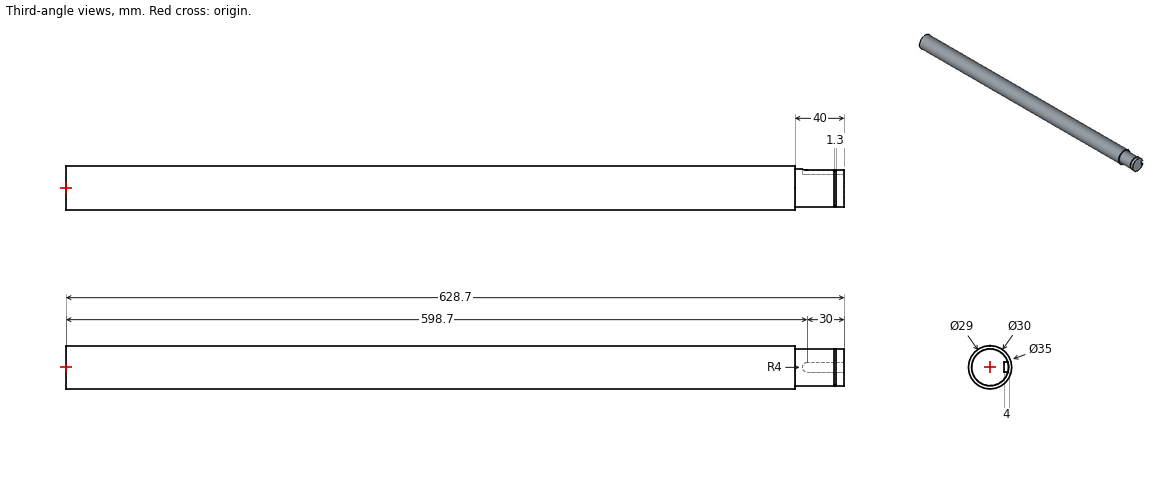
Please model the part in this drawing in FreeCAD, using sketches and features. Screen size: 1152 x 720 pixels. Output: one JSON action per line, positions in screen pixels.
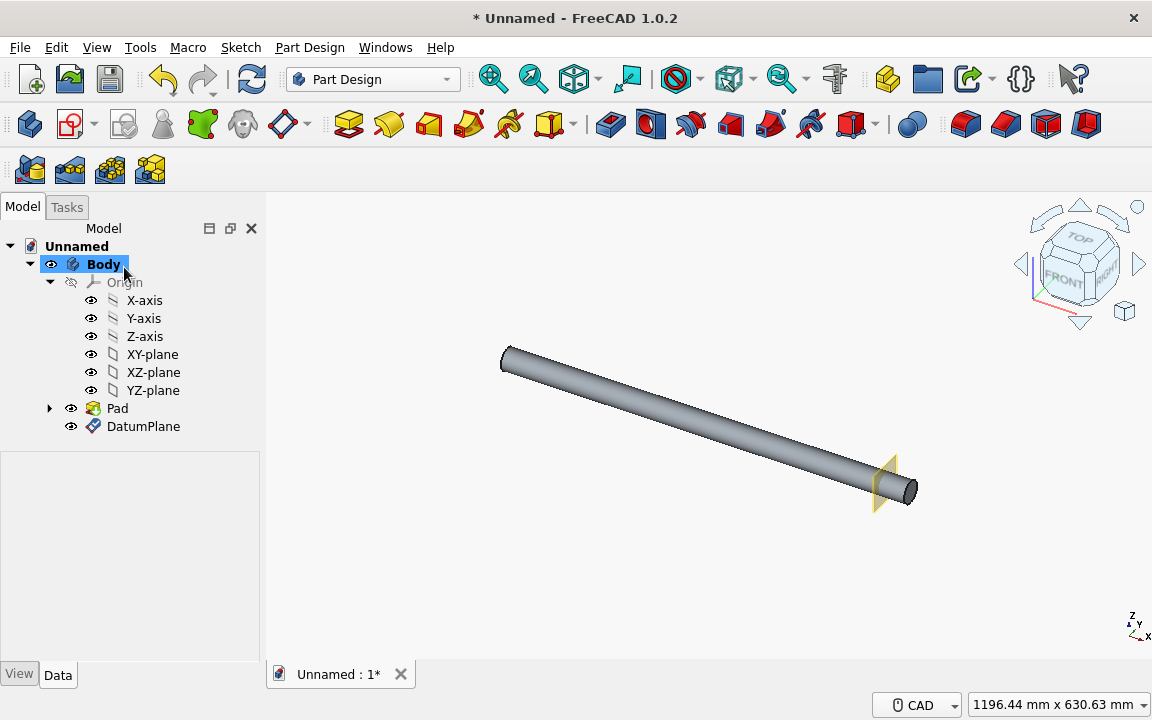
{"action": "left_click", "coordinate": [116, 426]}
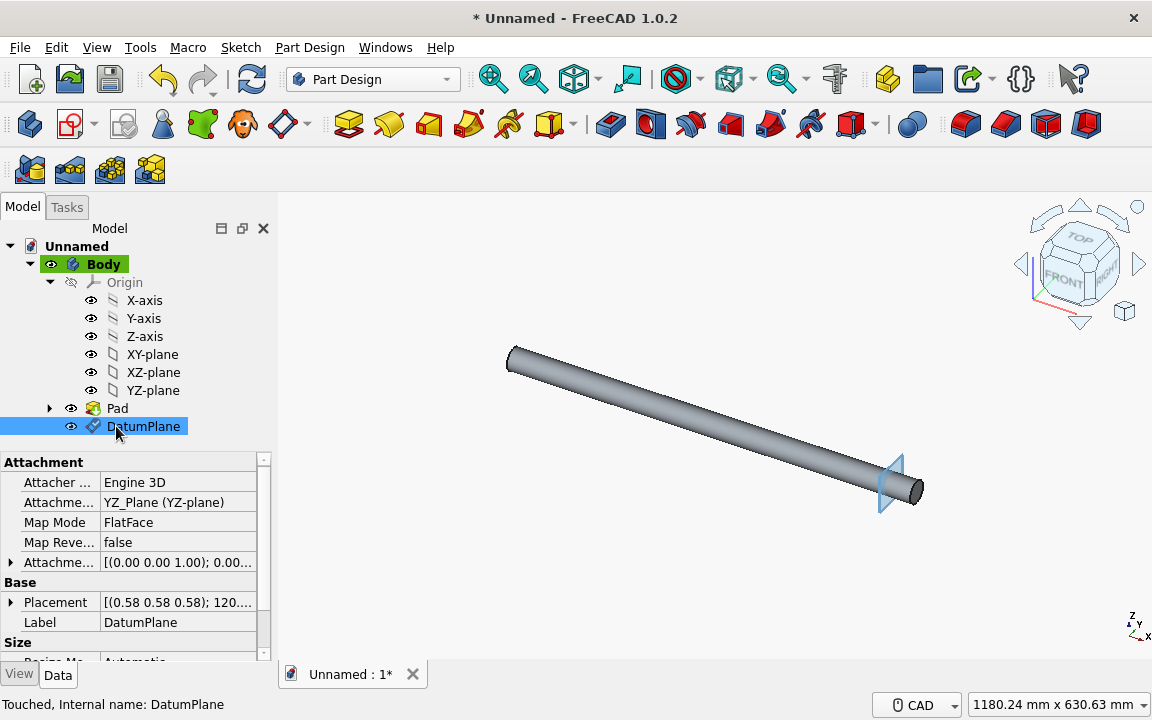
{"action": "left_click", "coordinate": [70, 124]}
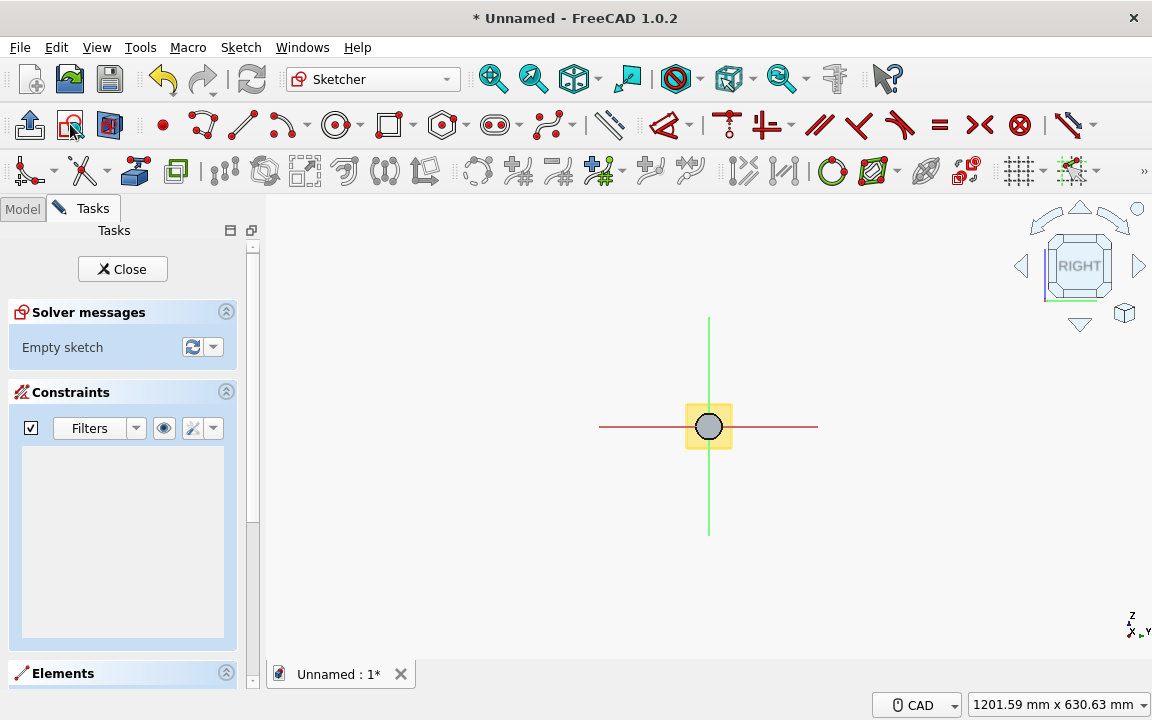
{"action": "key", "text": "q s"}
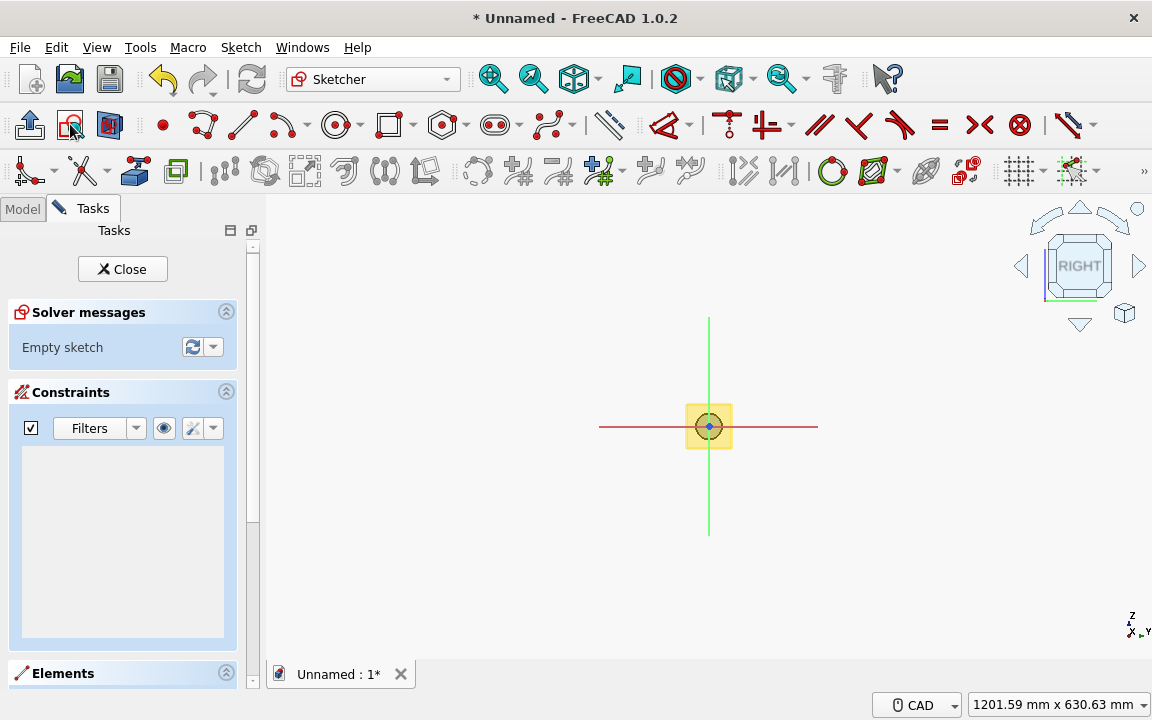
{"action": "scroll", "coordinate": [716, 426], "scroll_direction": "up", "scroll_amount": 12}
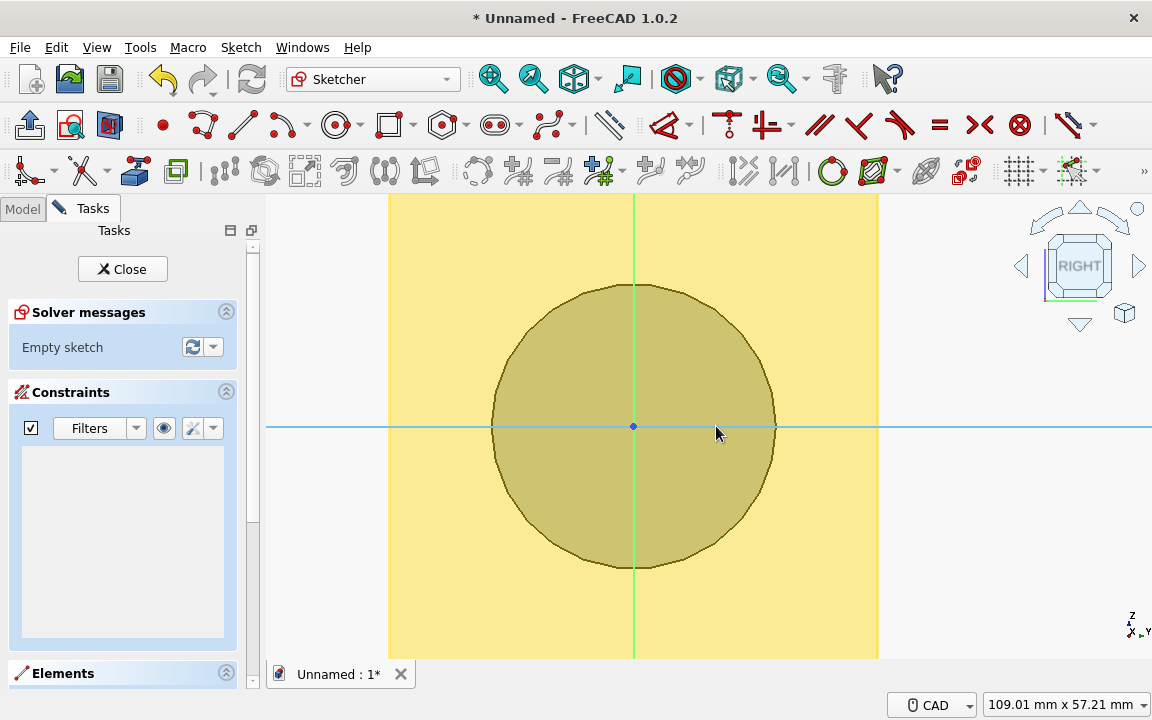
{"action": "left_click", "coordinate": [336, 126]}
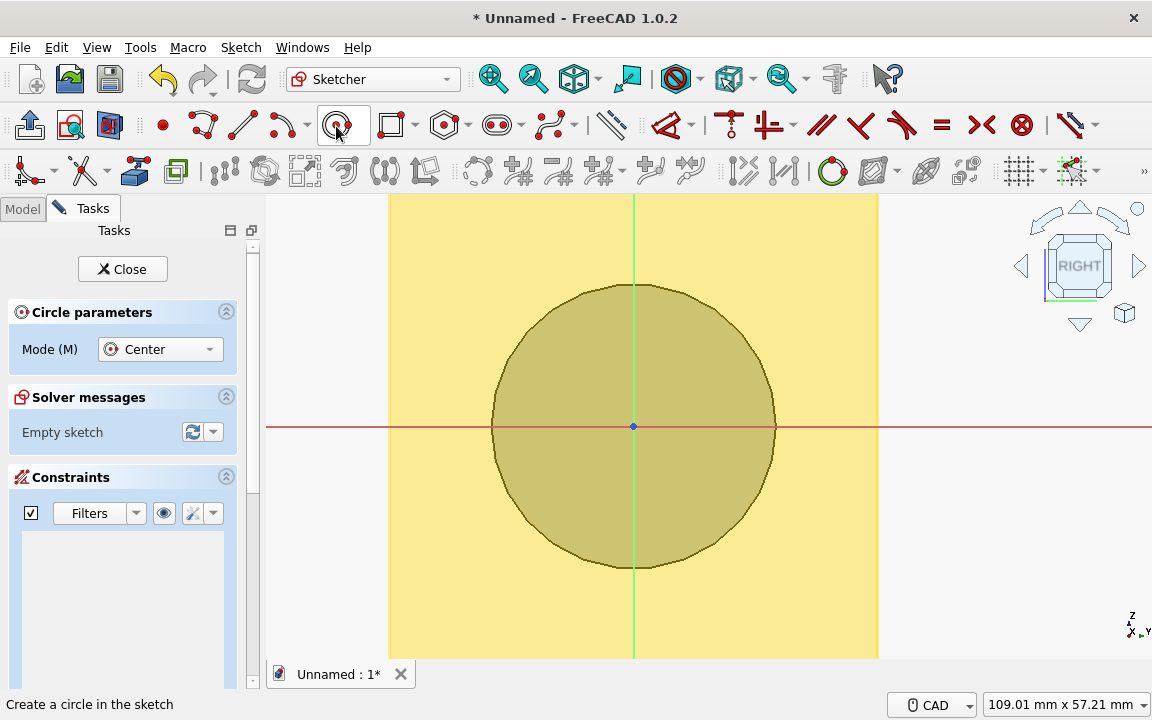
{"action": "left_click", "coordinate": [634, 426]}
{"action": "left_click", "coordinate": [734, 326]}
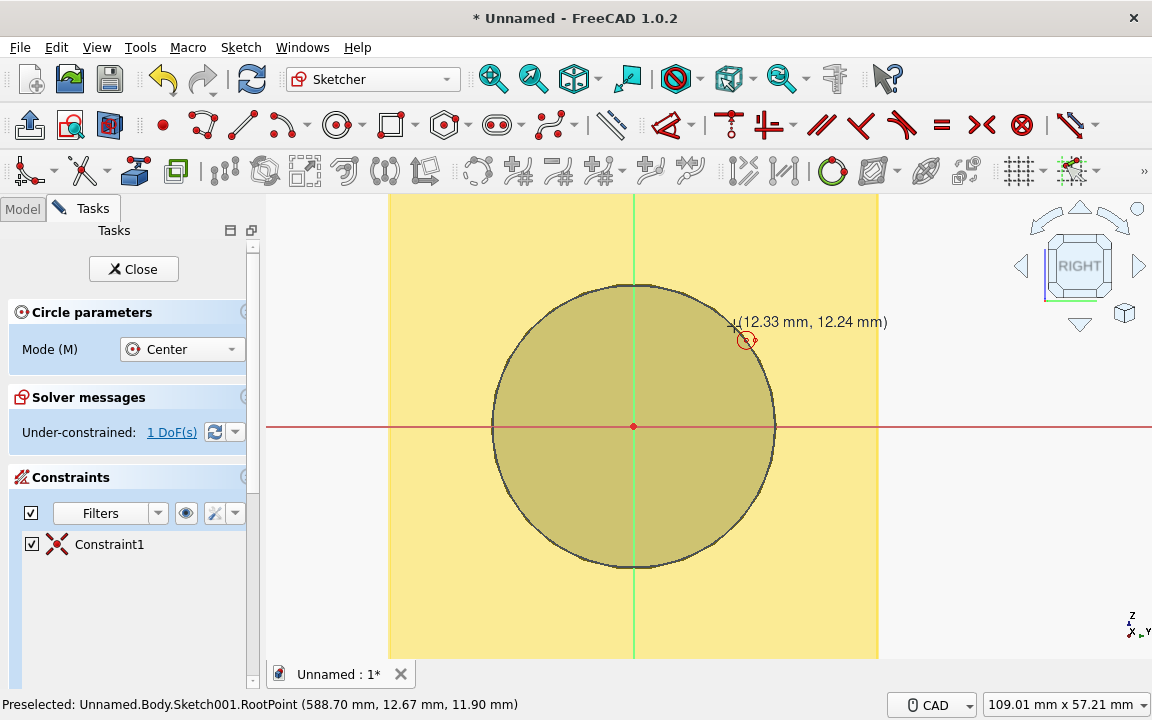
{"action": "left_click", "coordinate": [634, 426]}
{"action": "left_click", "coordinate": [720, 340]}
{"action": "key", "text": "Escape"}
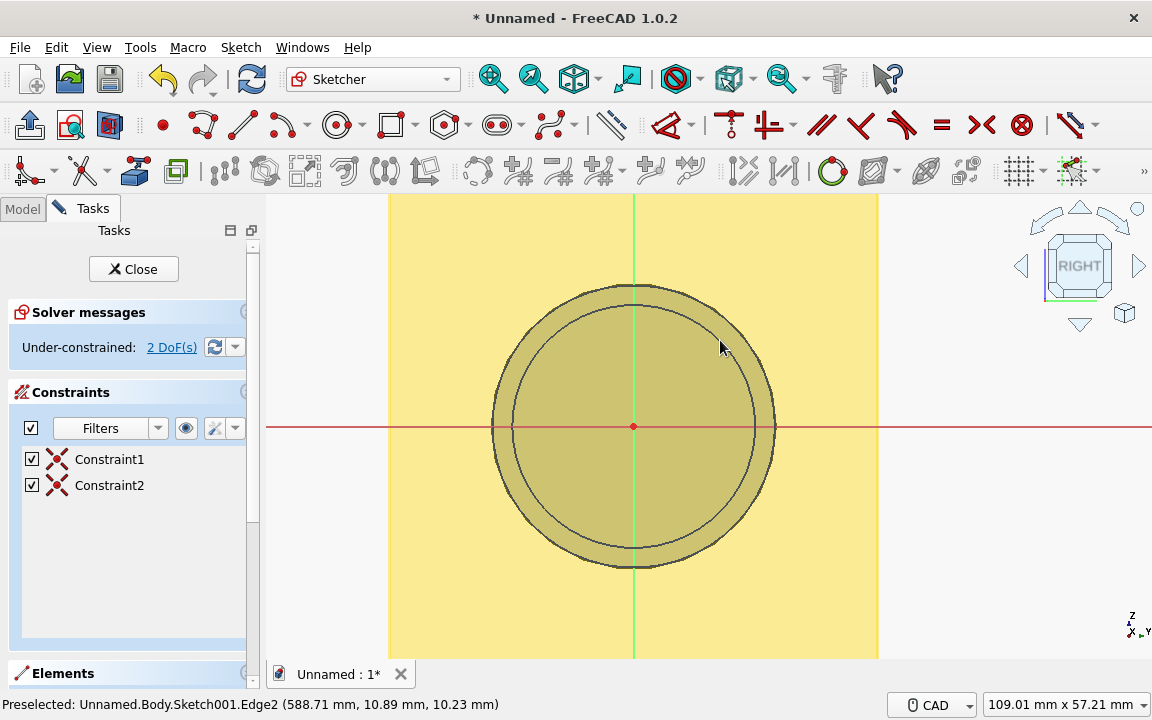
{"action": "left_click", "coordinate": [666, 126]}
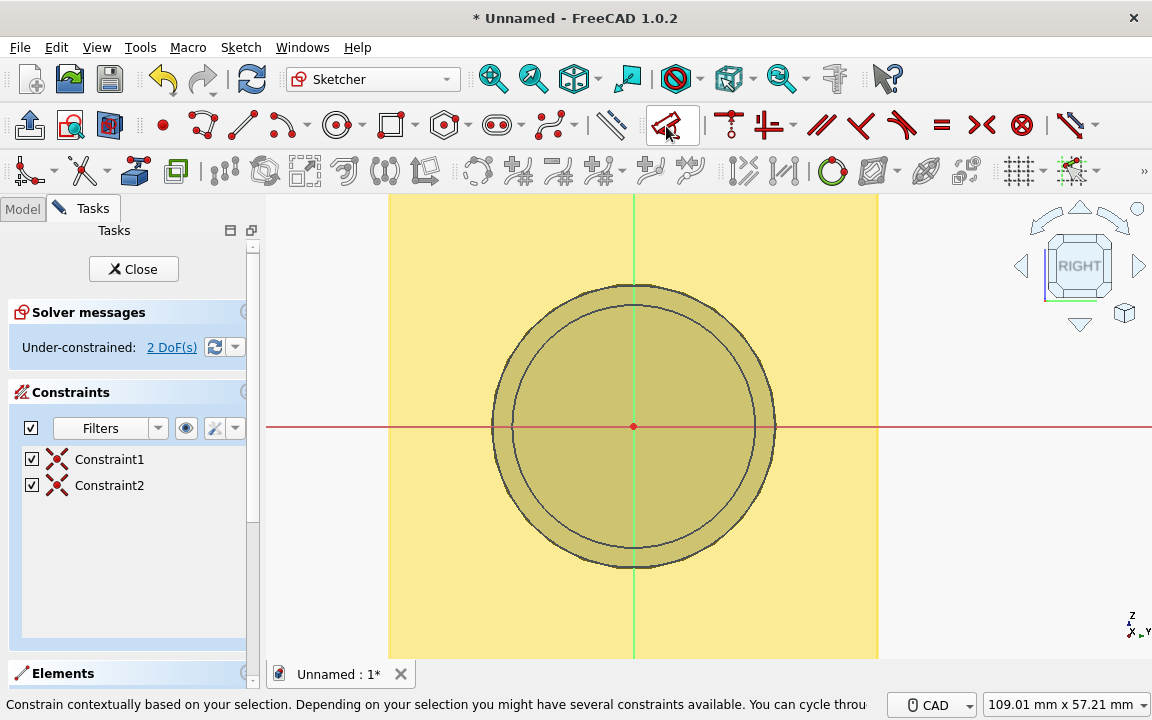
{"action": "left_click", "coordinate": [733, 326]}
{"action": "left_click", "coordinate": [755, 303]}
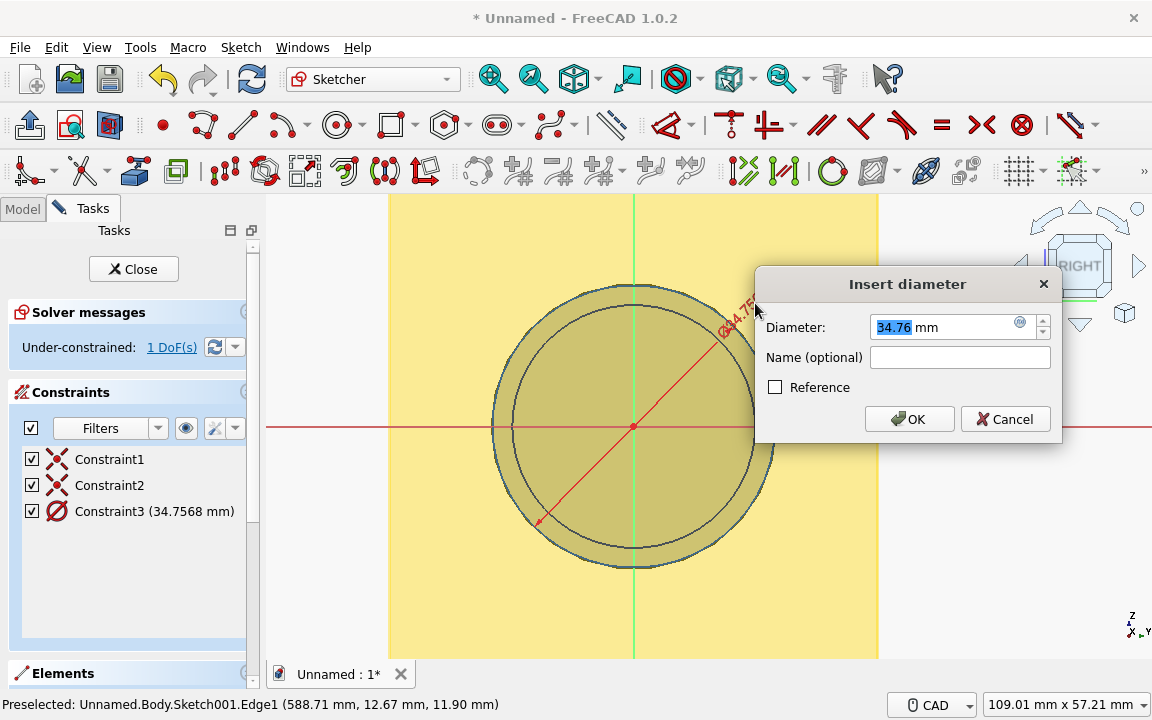
{"action": "type", "text": "35"}
{"action": "key", "text": "Return"}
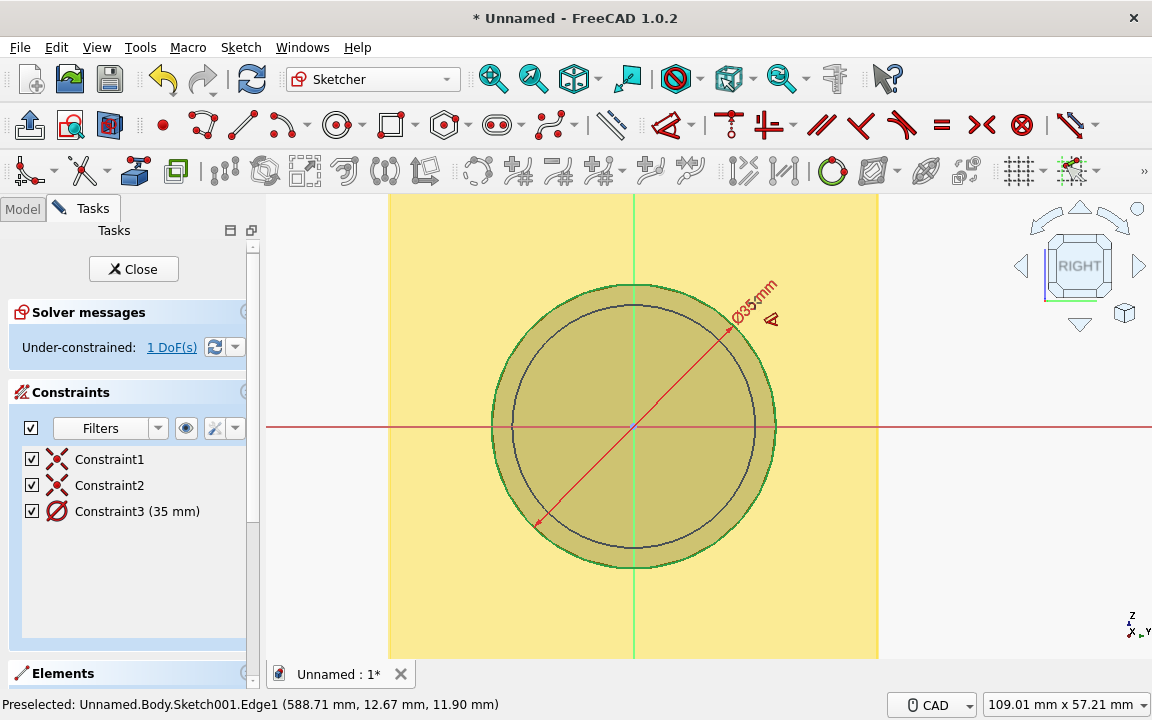
{"action": "left_click", "coordinate": [719, 340]}
{"action": "left_click", "coordinate": [803, 376]}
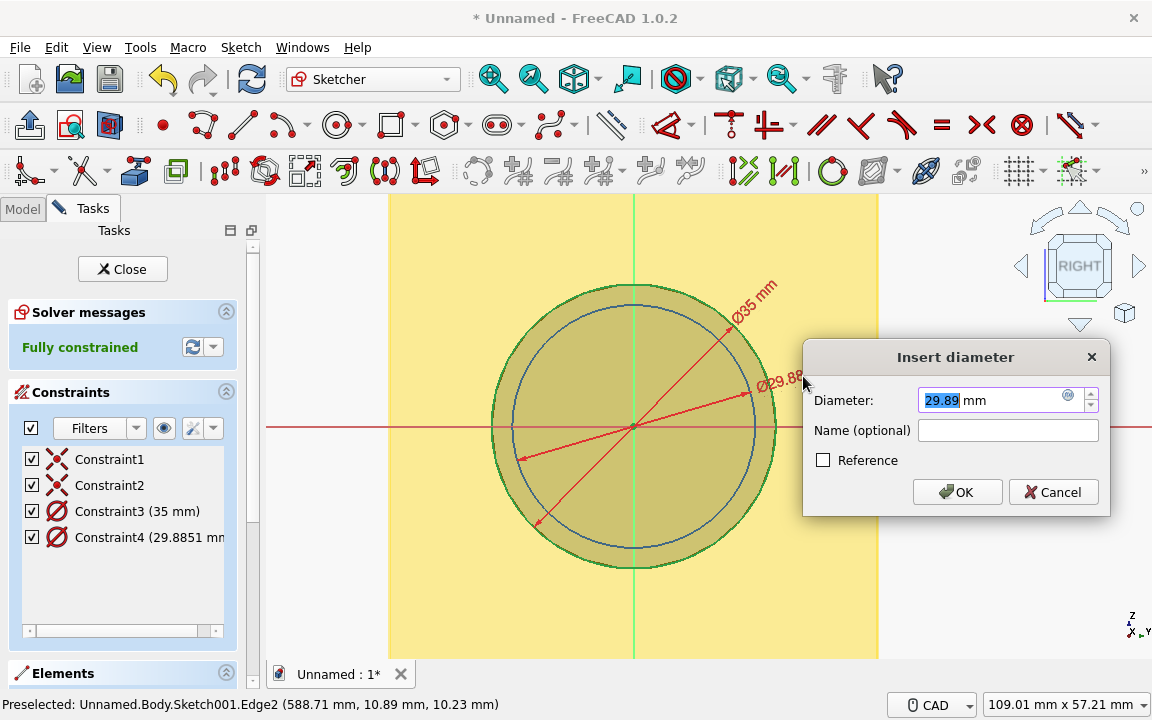
{"action": "type", "text": "30"}
{"action": "key", "text": "Return"}
{"action": "key", "text": "Escape"}